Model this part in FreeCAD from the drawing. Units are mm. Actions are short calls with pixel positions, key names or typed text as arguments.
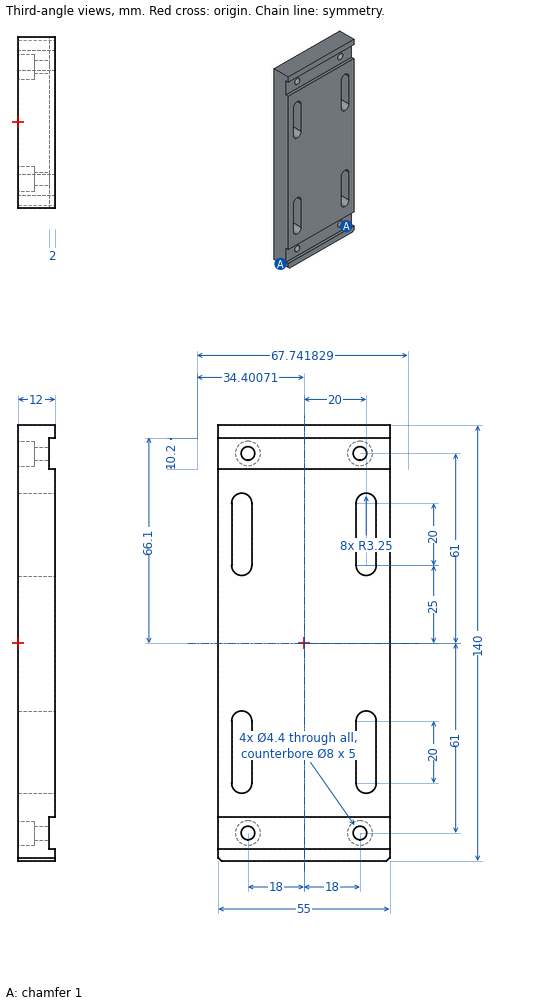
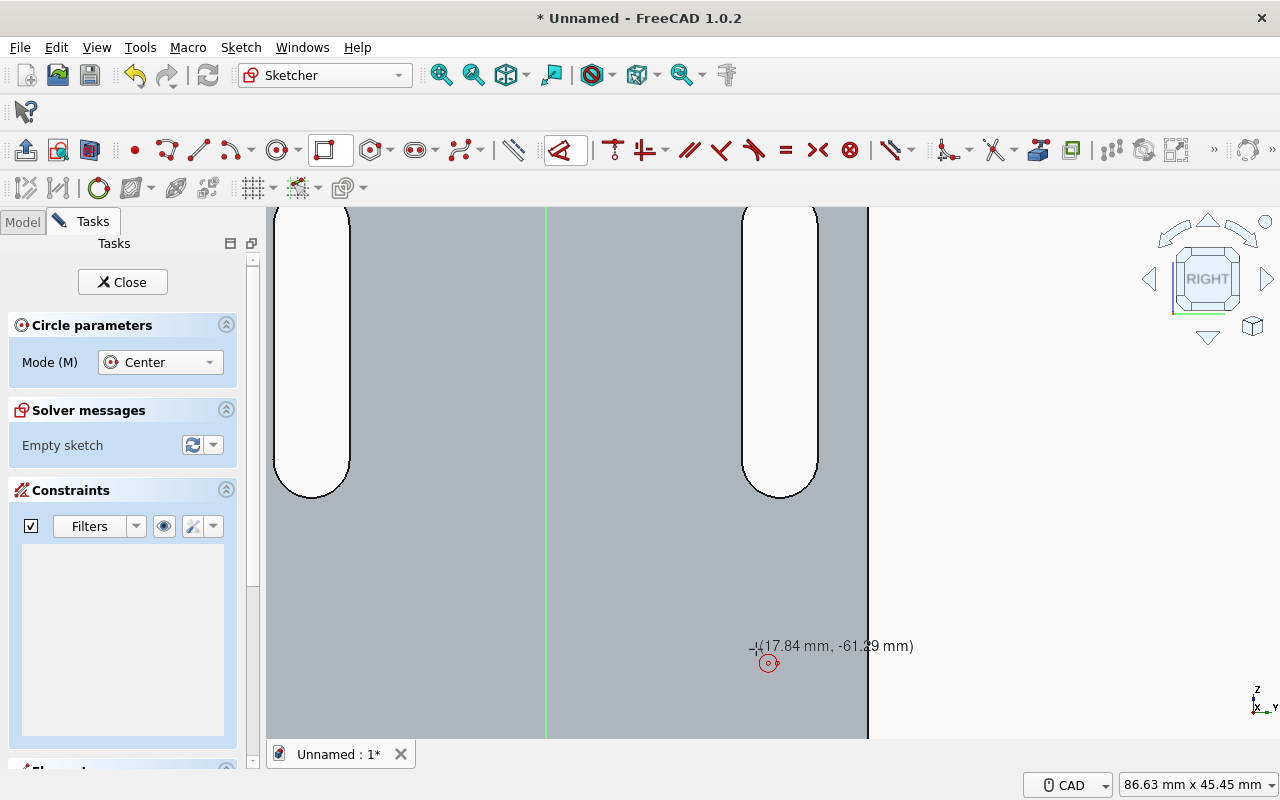
scroll(756, 650, down, 7)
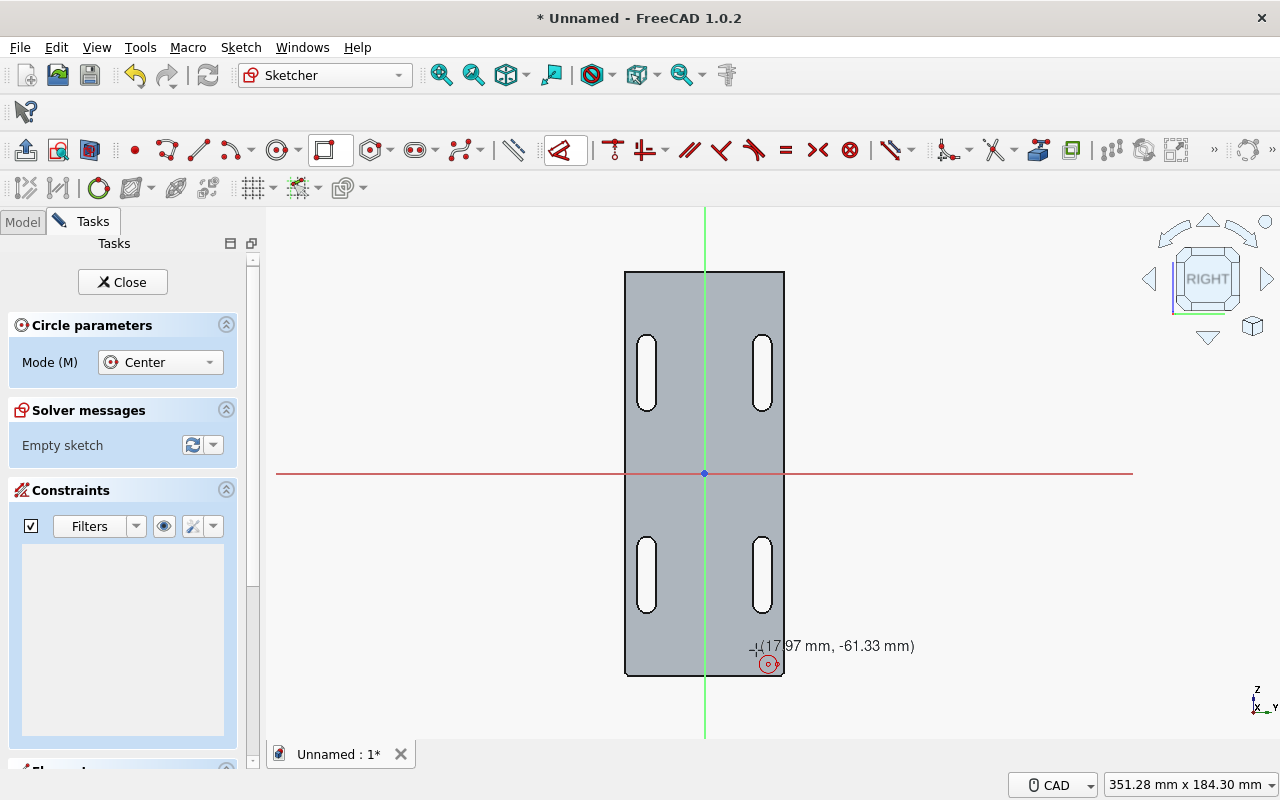
click(756, 650)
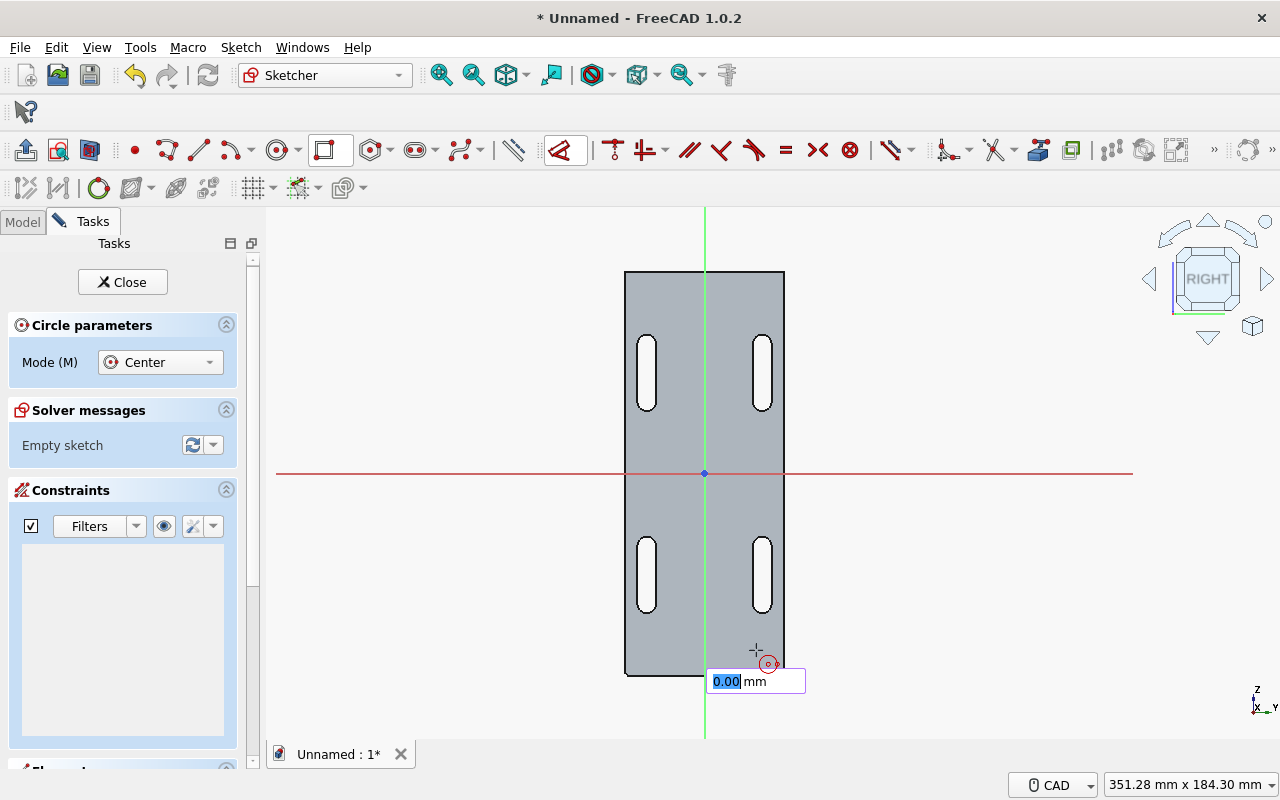
scroll(761, 645, up, 5)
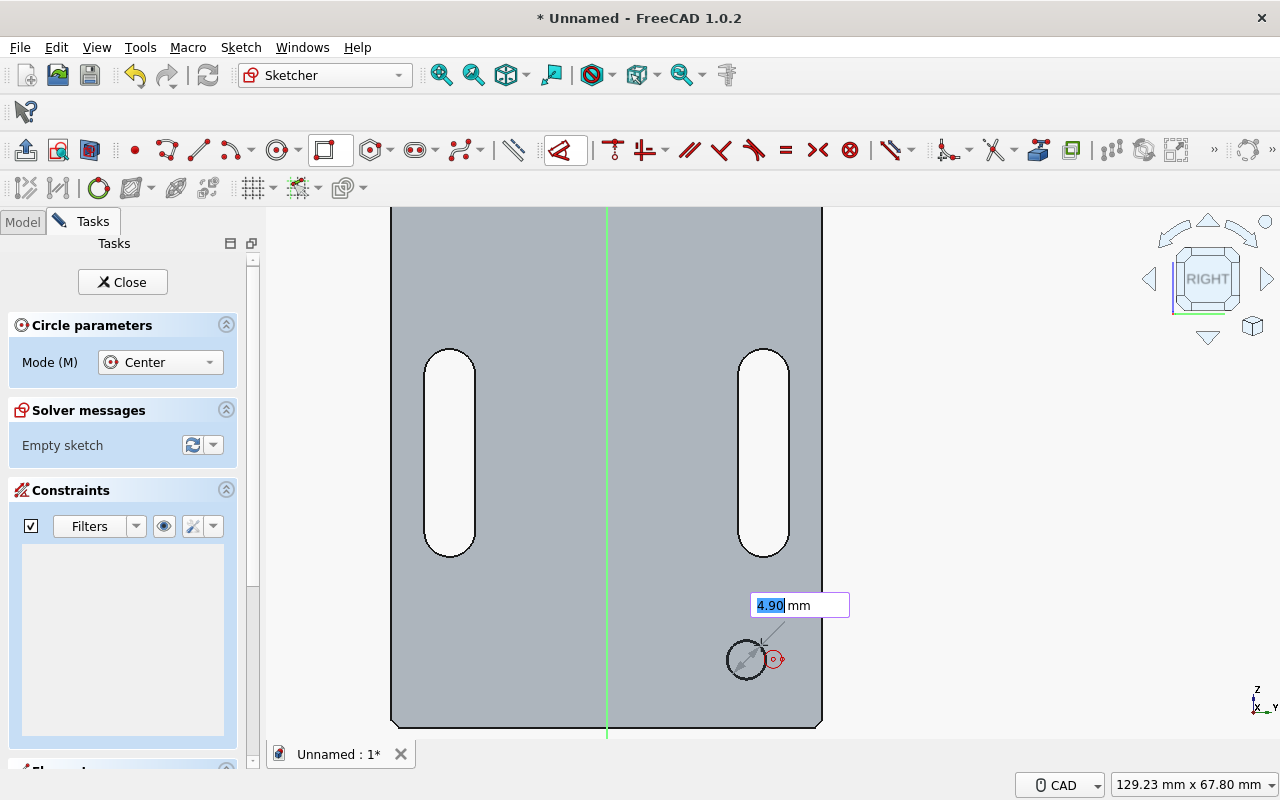
click(760, 645)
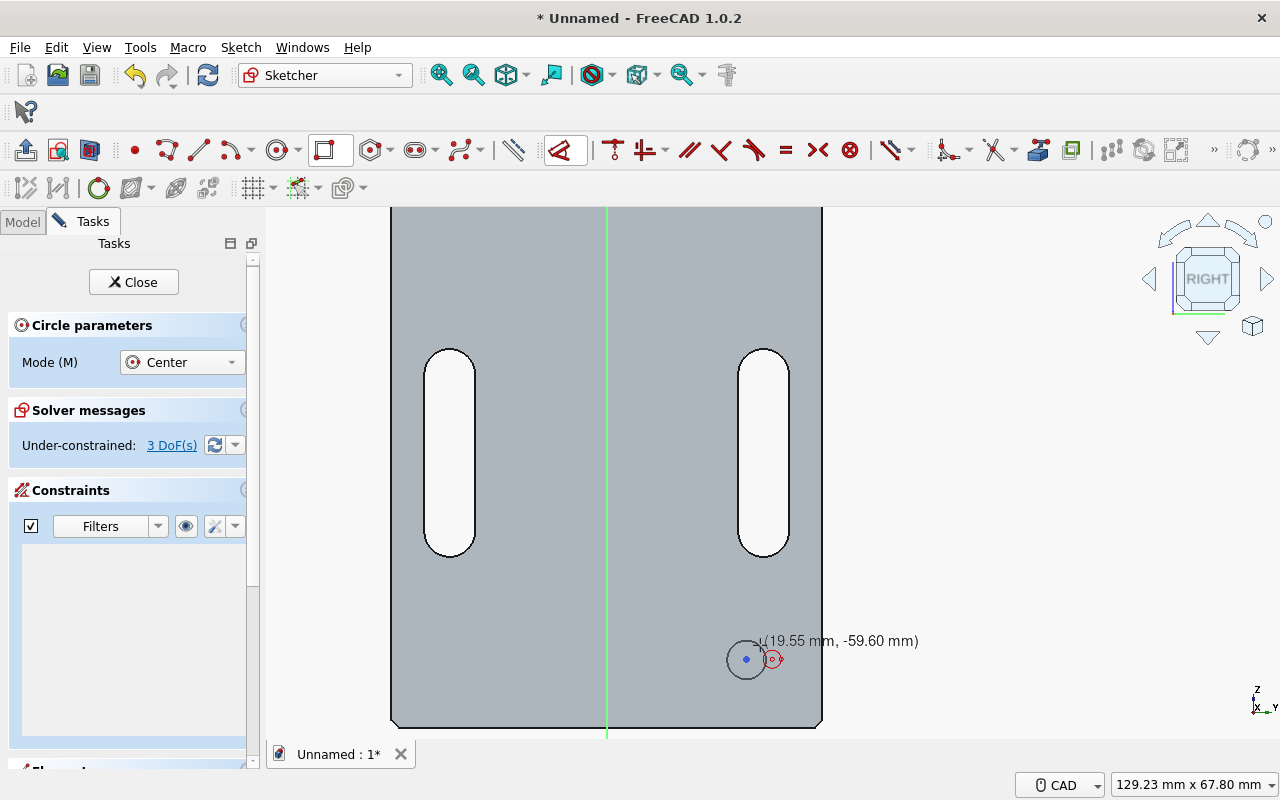
scroll(465, 657, up, 2)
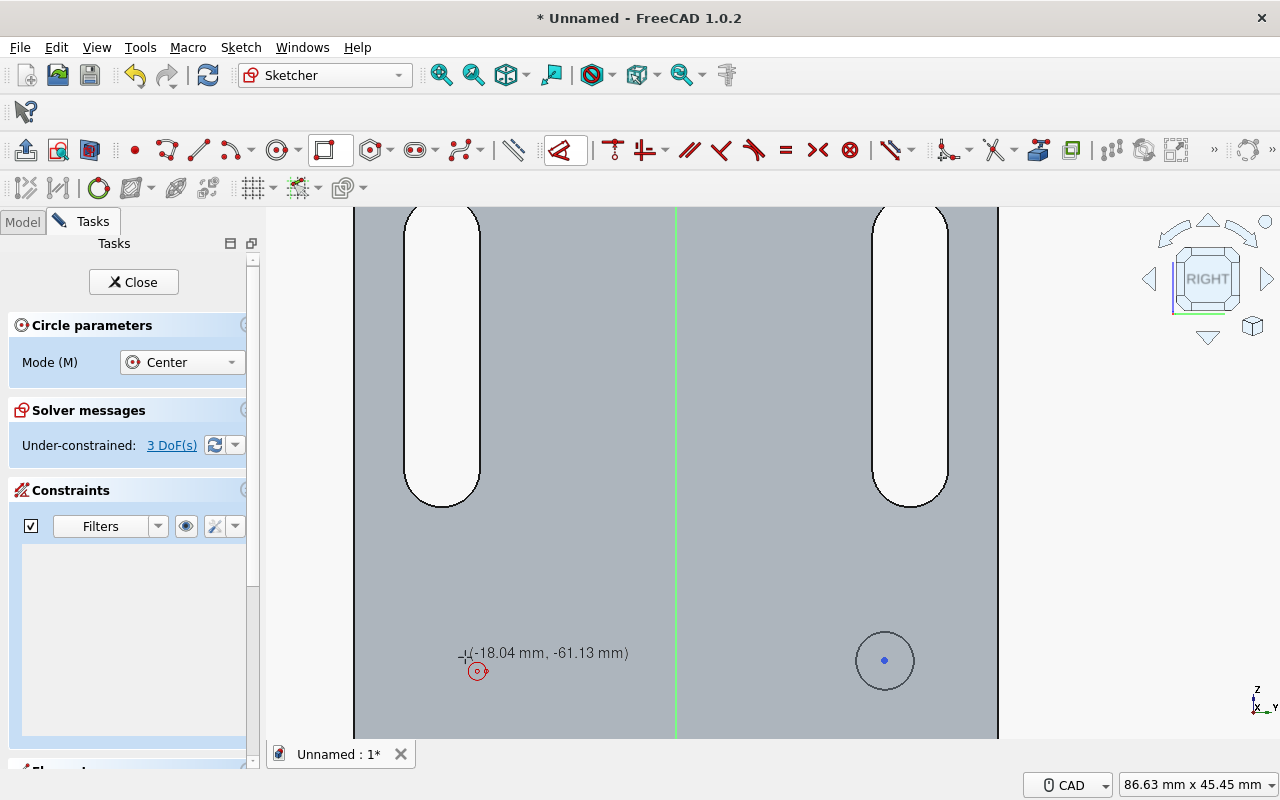
scroll(714, 647, down, 7)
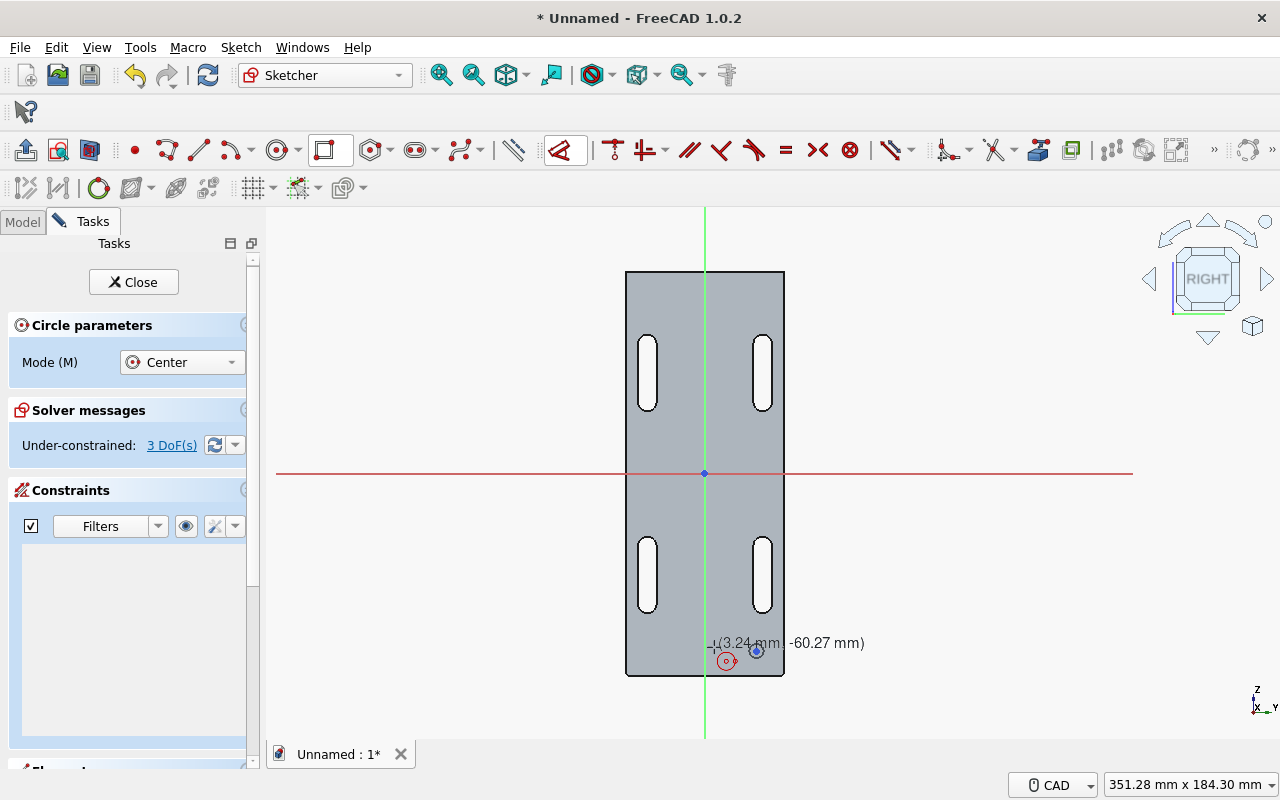
click(653, 650)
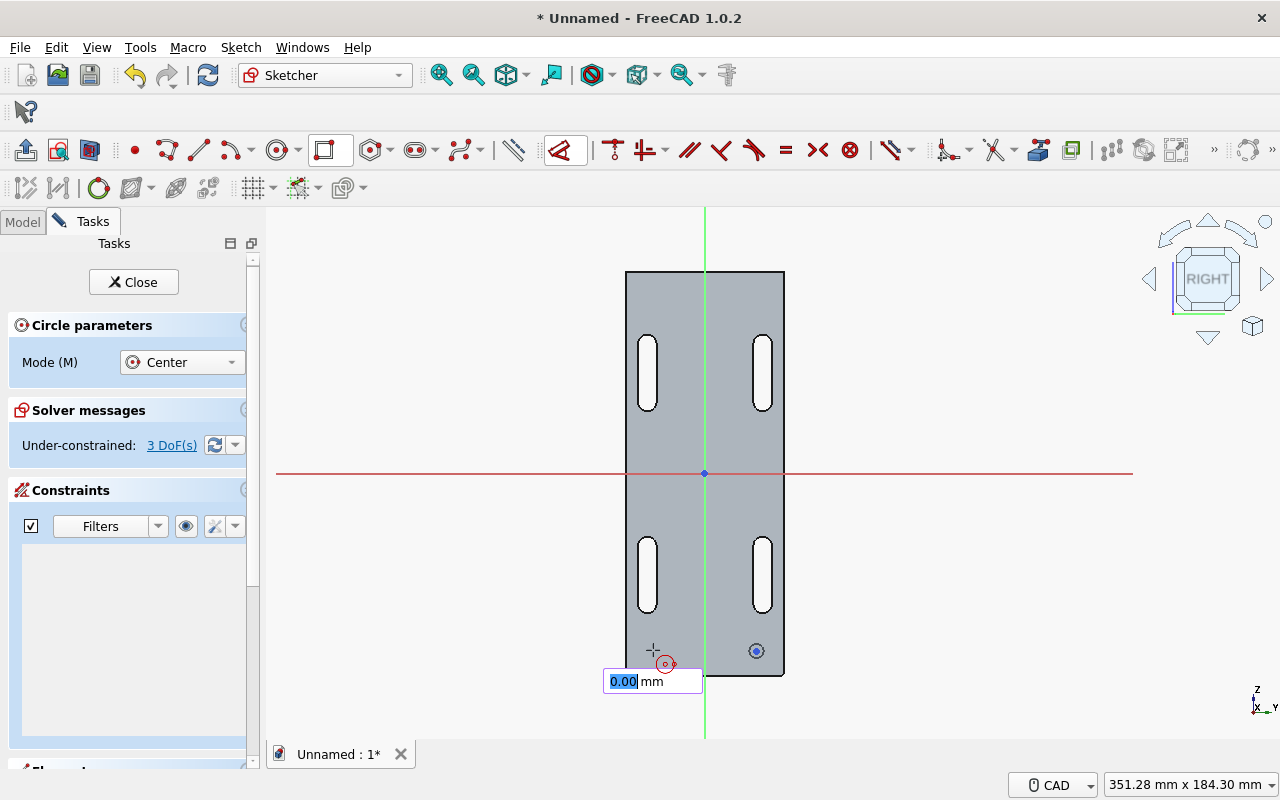
scroll(658, 645, up, 5)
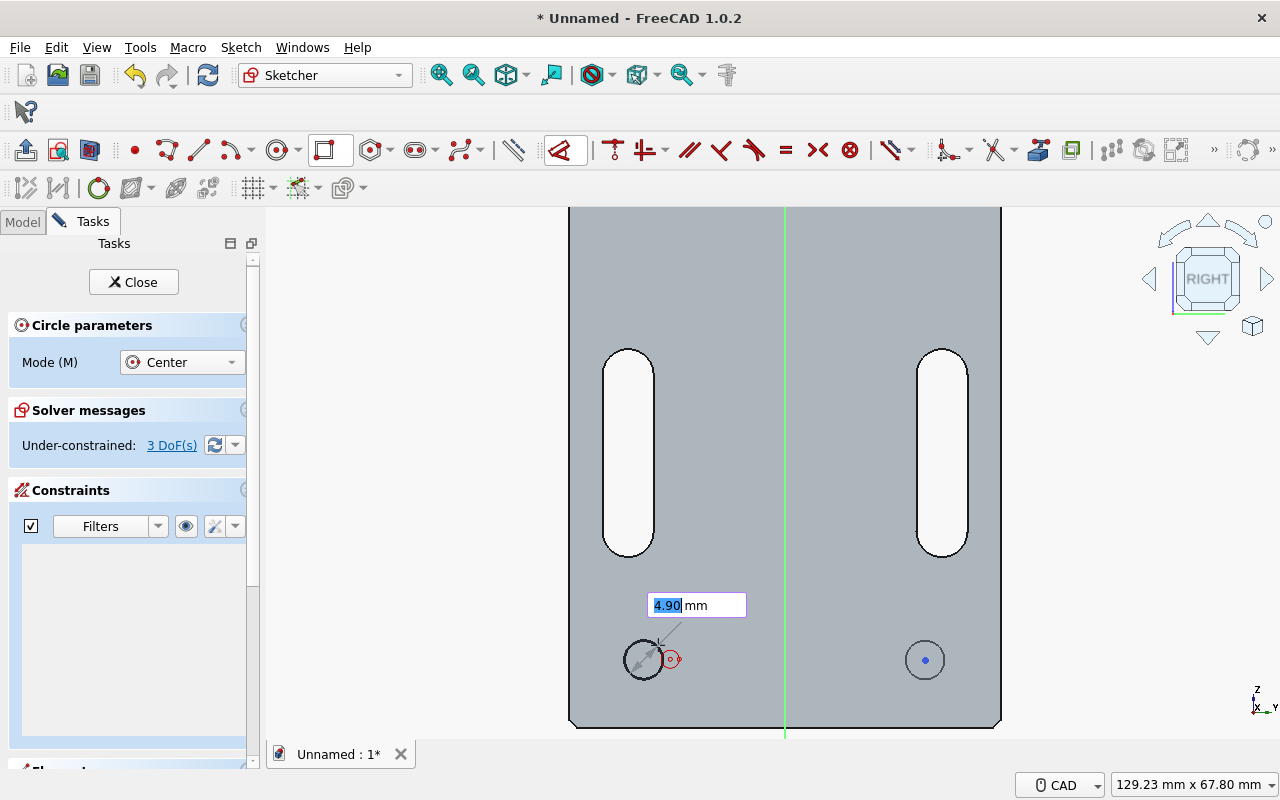
click(656, 645)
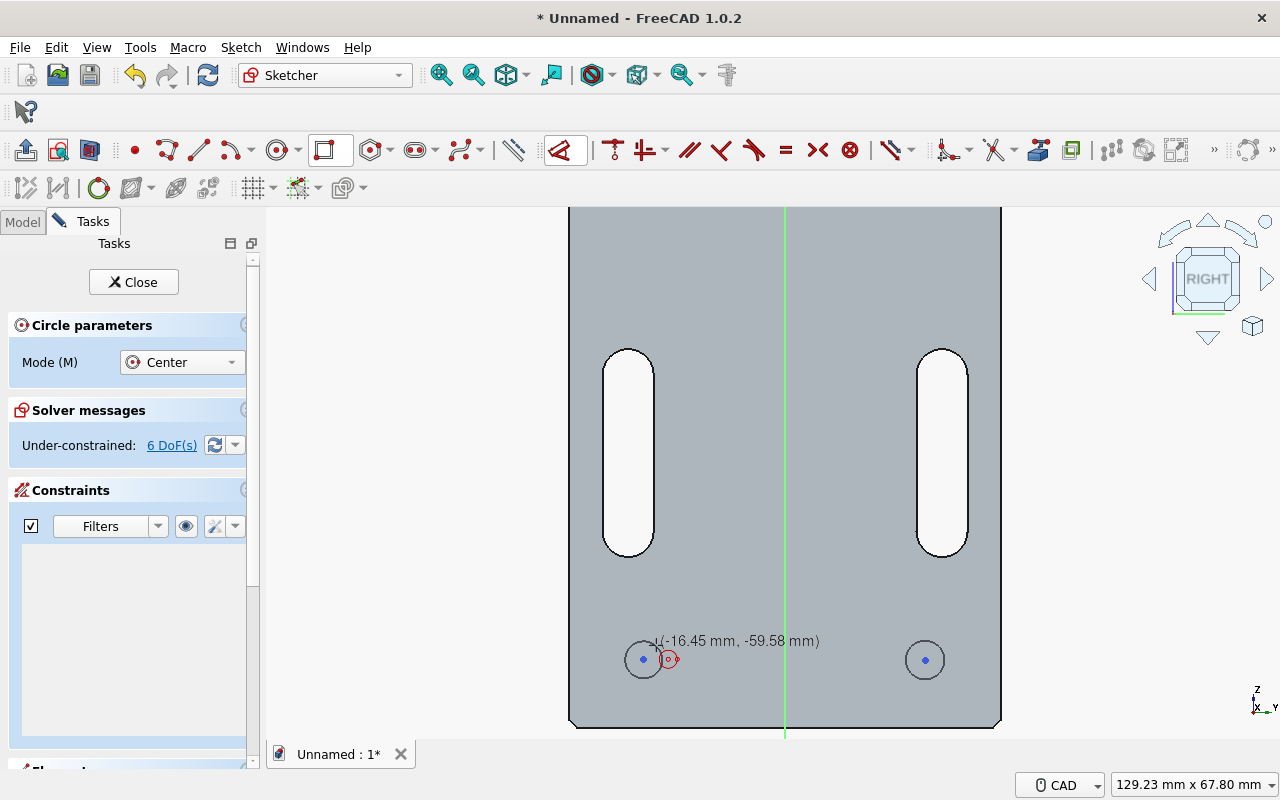
scroll(658, 644, down, 5)